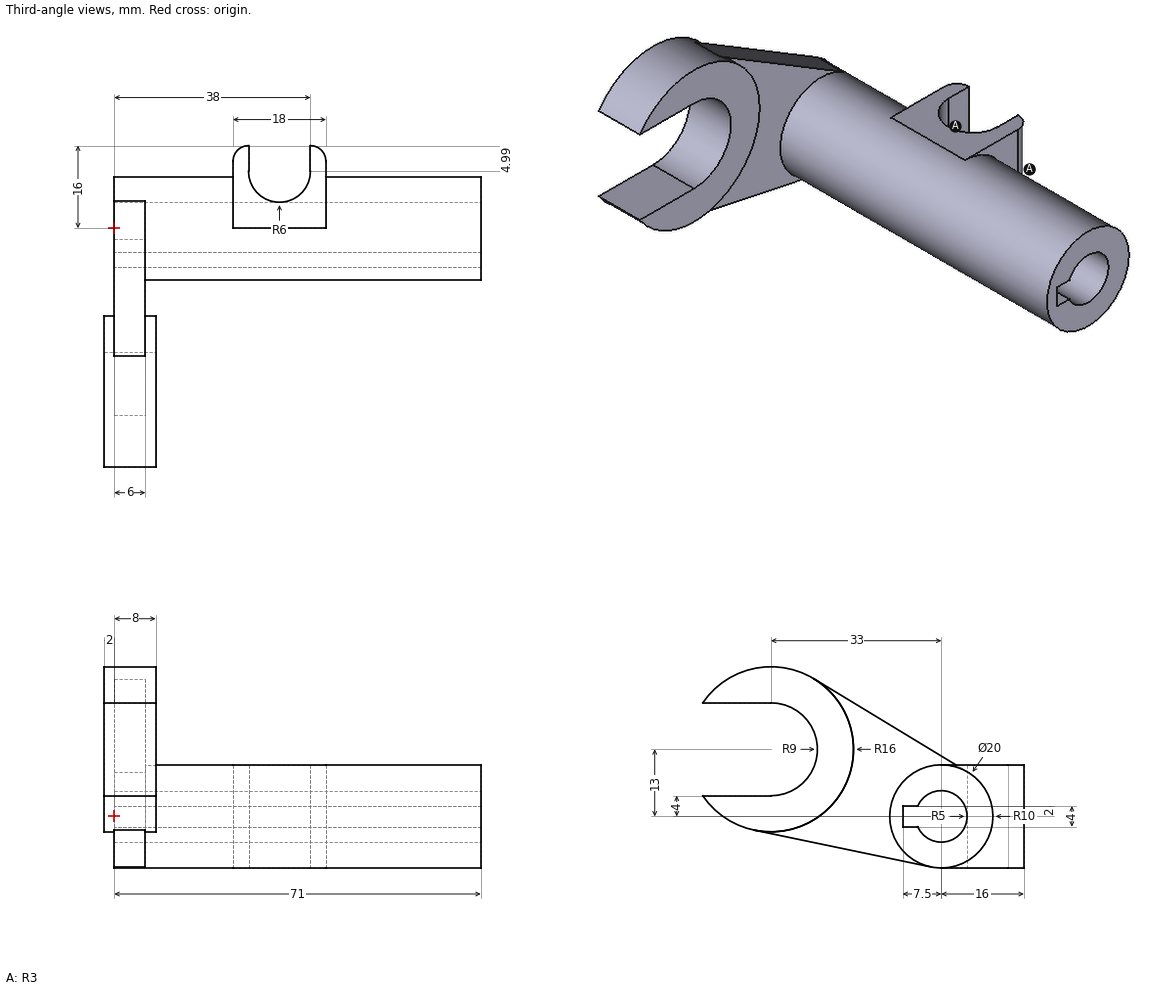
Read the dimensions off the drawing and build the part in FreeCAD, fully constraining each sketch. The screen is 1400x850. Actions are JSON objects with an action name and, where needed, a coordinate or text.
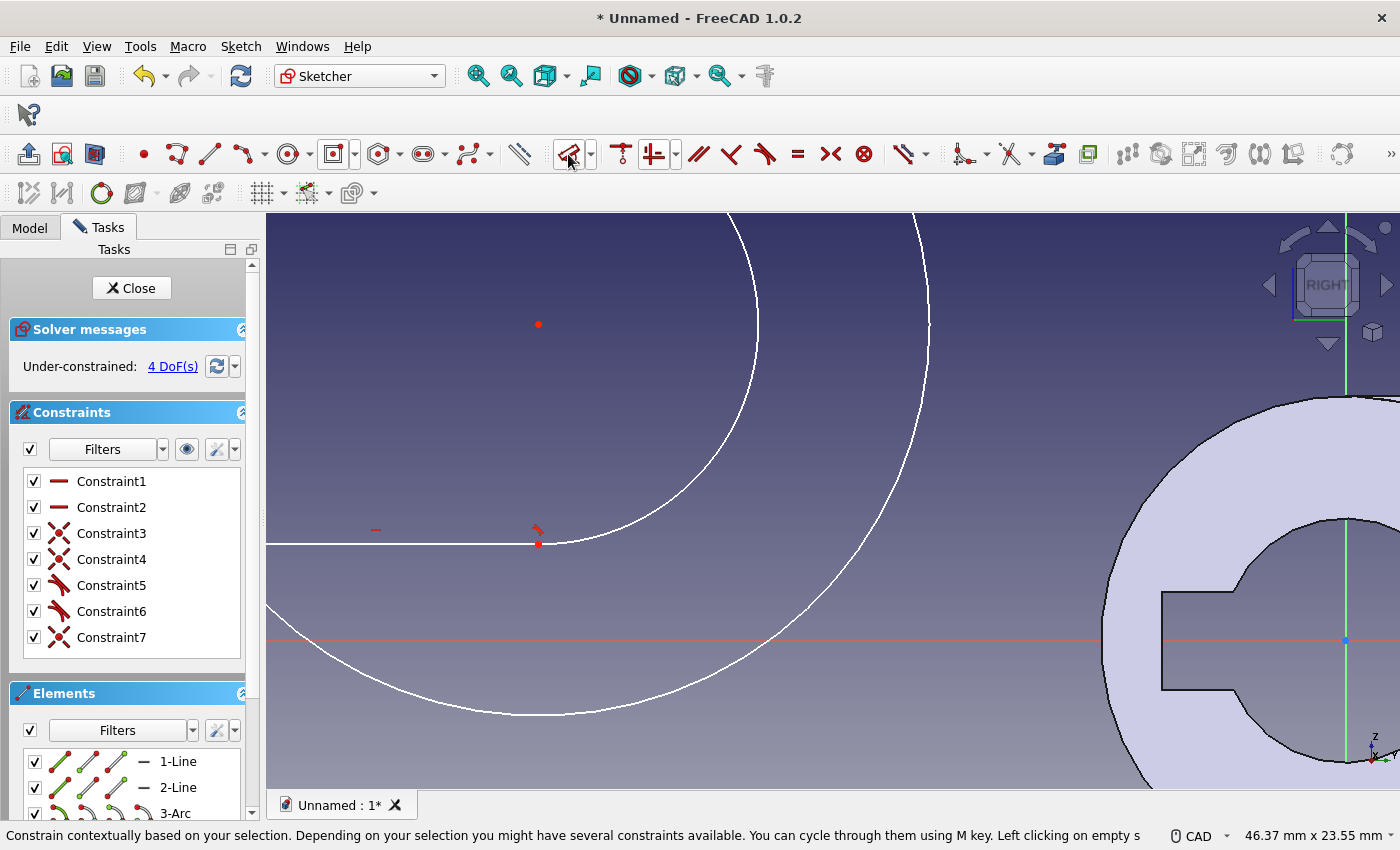
{"action": "left_click", "coordinate": [744, 658]}
{"action": "left_click", "coordinate": [761, 685]}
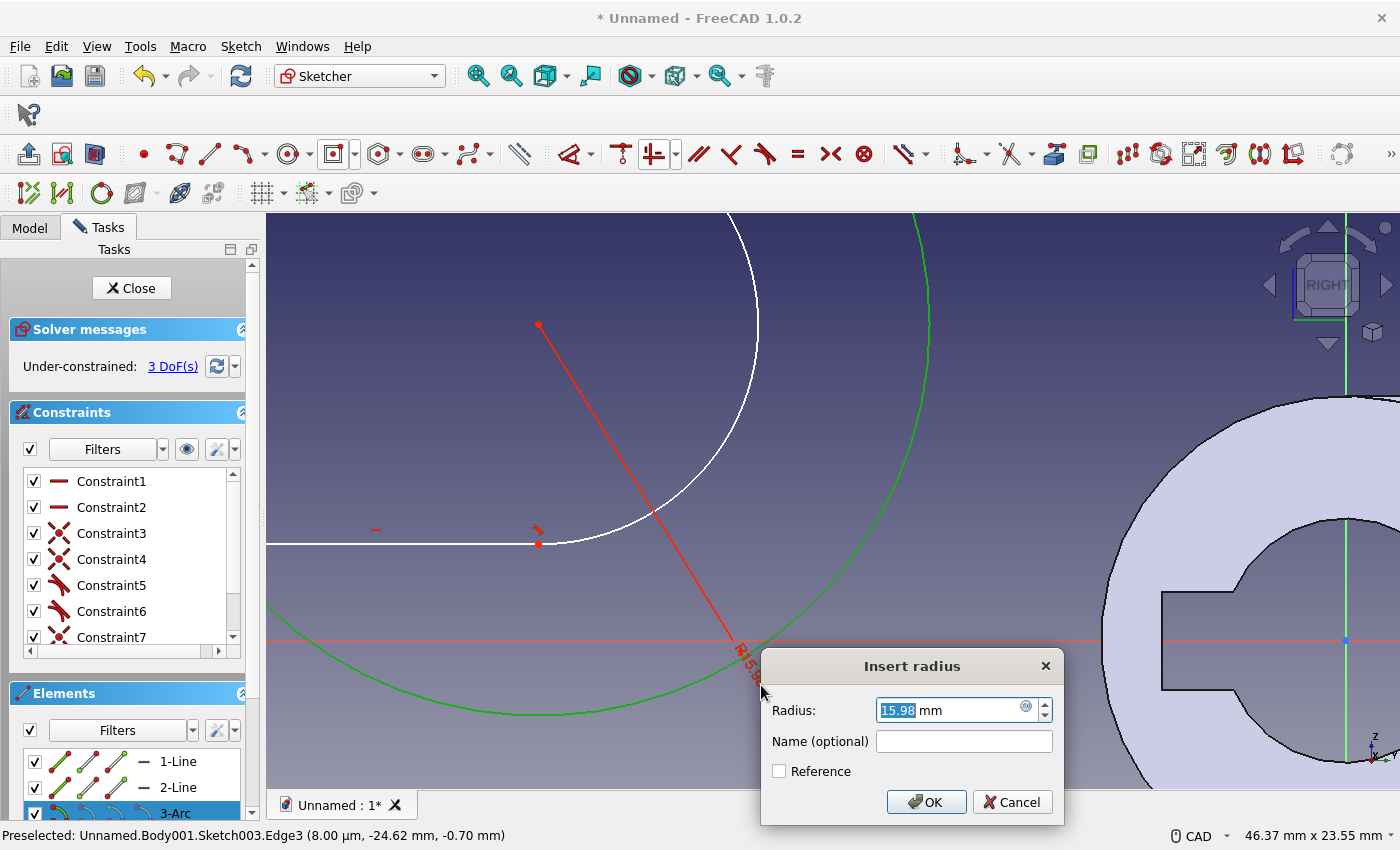
{"action": "type", "text": "16"}
{"action": "key", "text": "Return"}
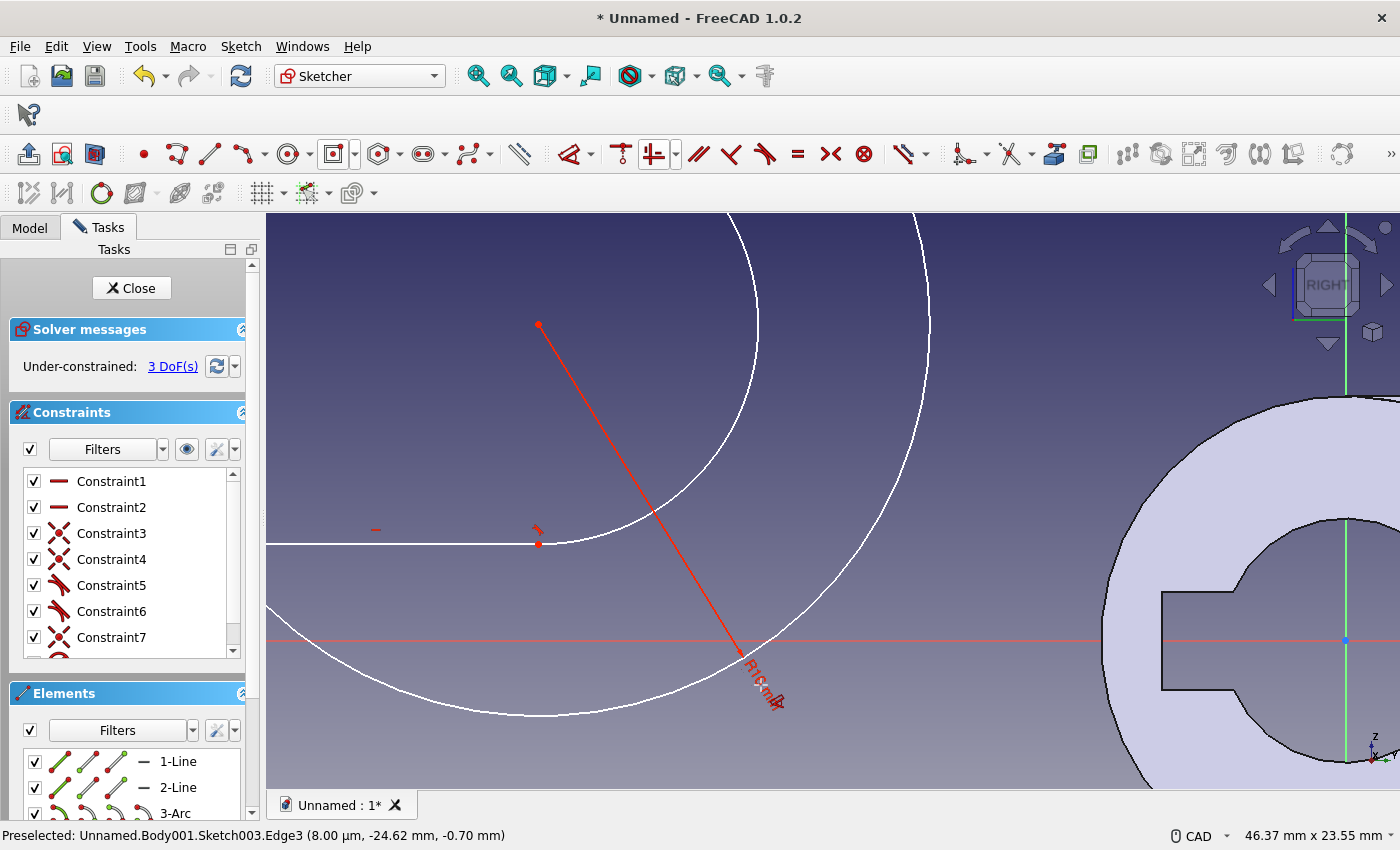
{"action": "left_click", "coordinate": [716, 454]}
{"action": "left_click", "coordinate": [742, 473]}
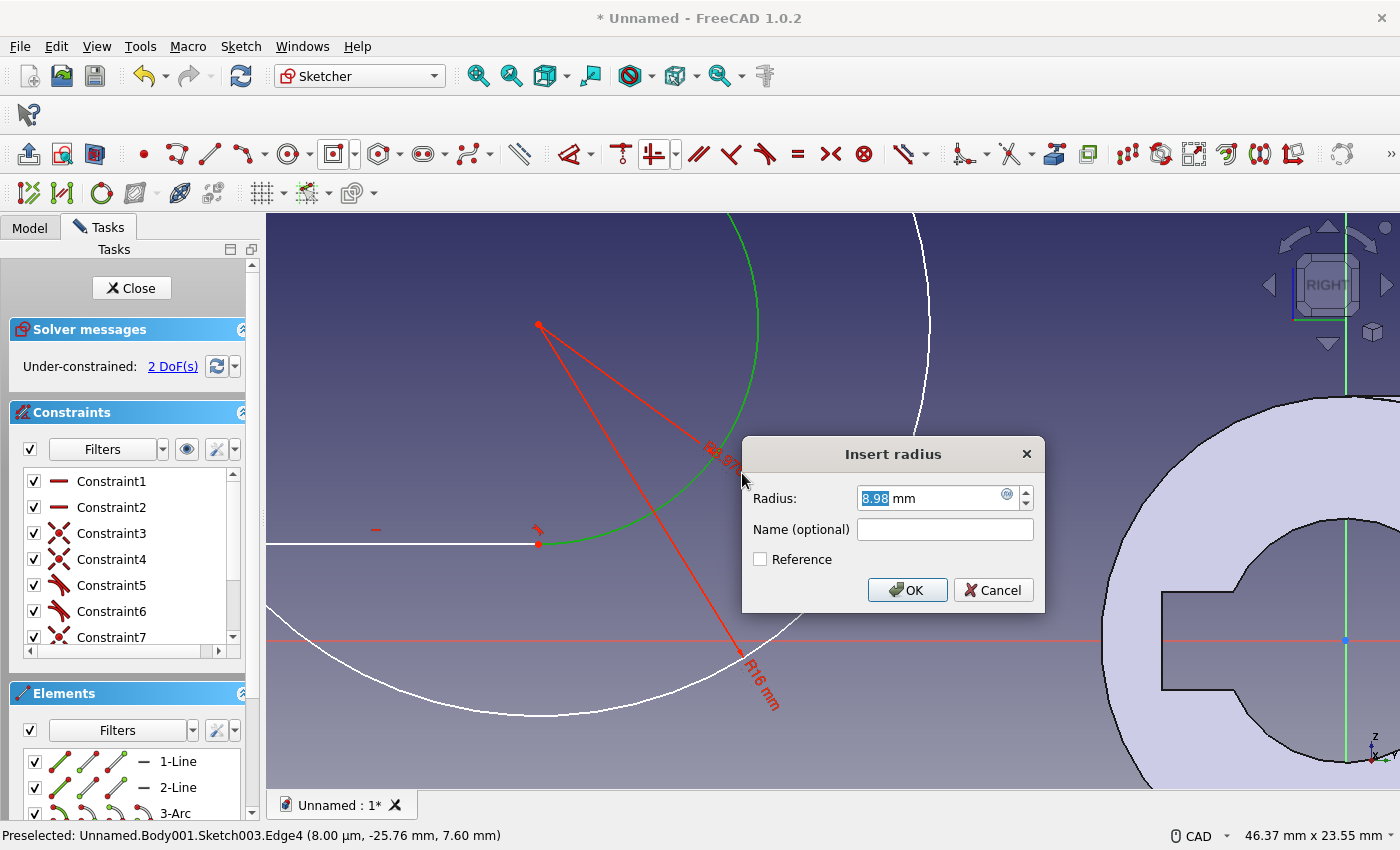
{"action": "type", "text": "9"}
{"action": "key", "text": "Return"}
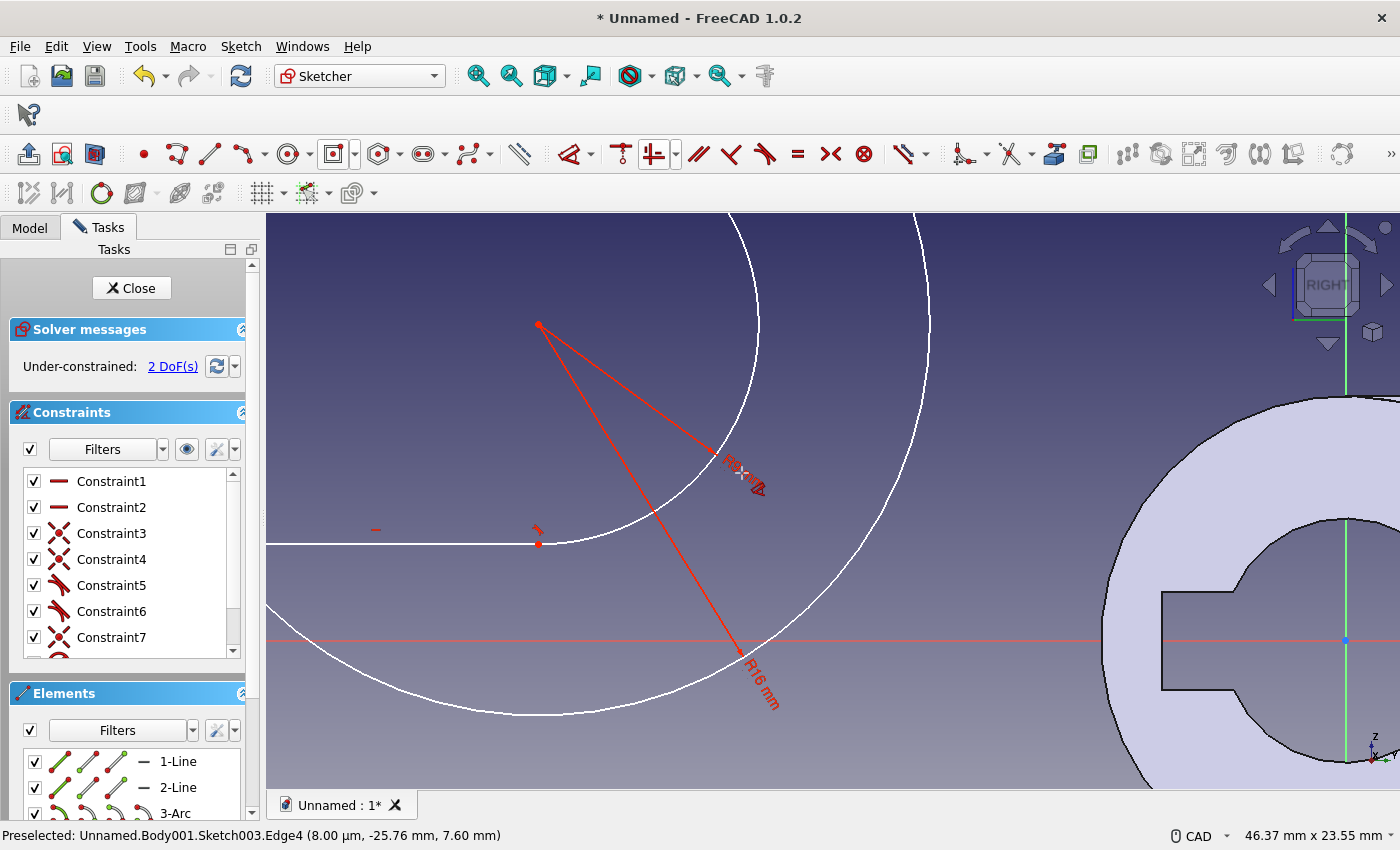
{"action": "scroll", "coordinate": [745, 658], "scroll_direction": "down", "scroll_amount": 3}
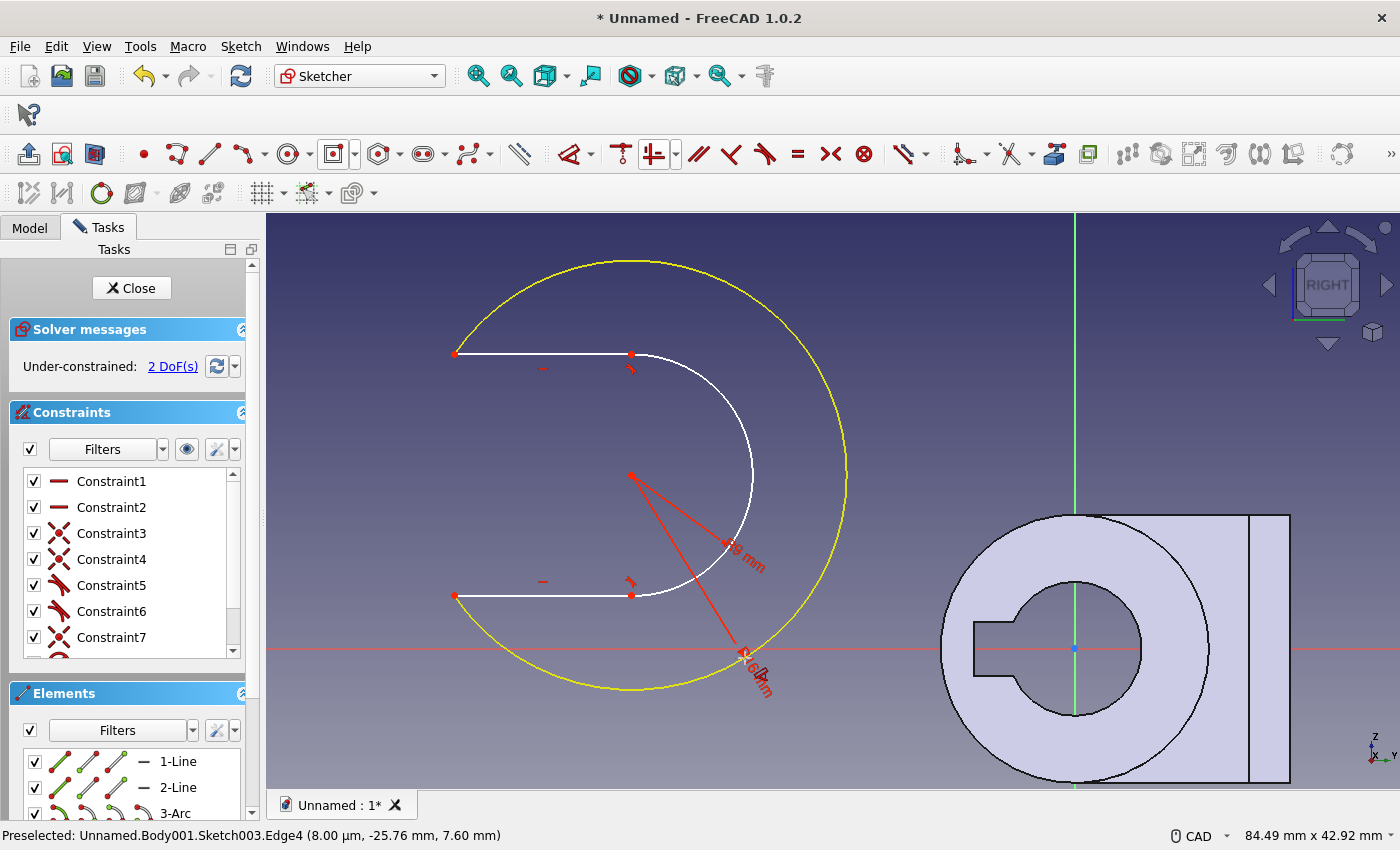
{"action": "left_click", "coordinate": [454, 596]}
{"action": "left_click", "coordinate": [1109, 622]}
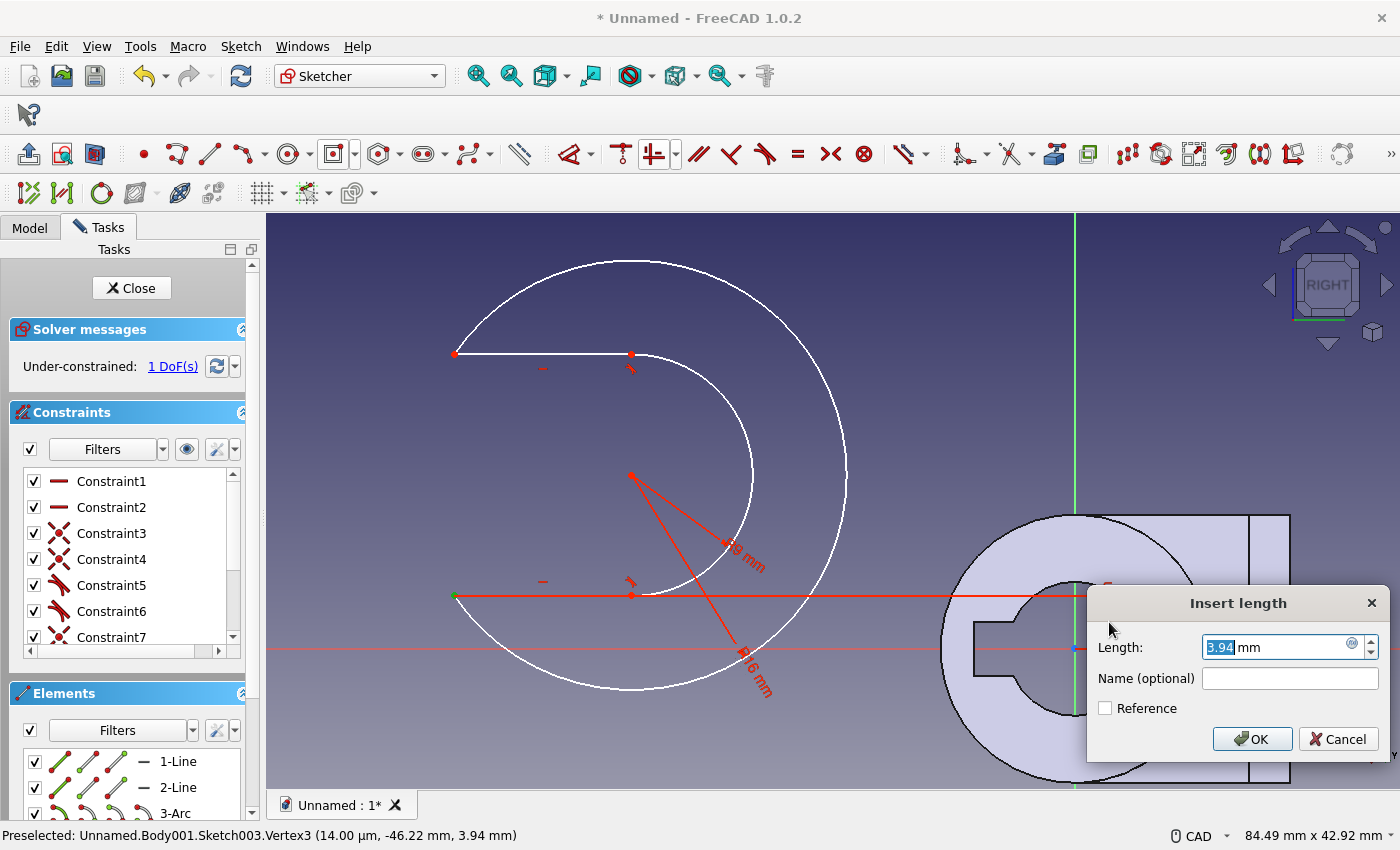
{"action": "type", "text": "4"}
{"action": "key", "text": "Return"}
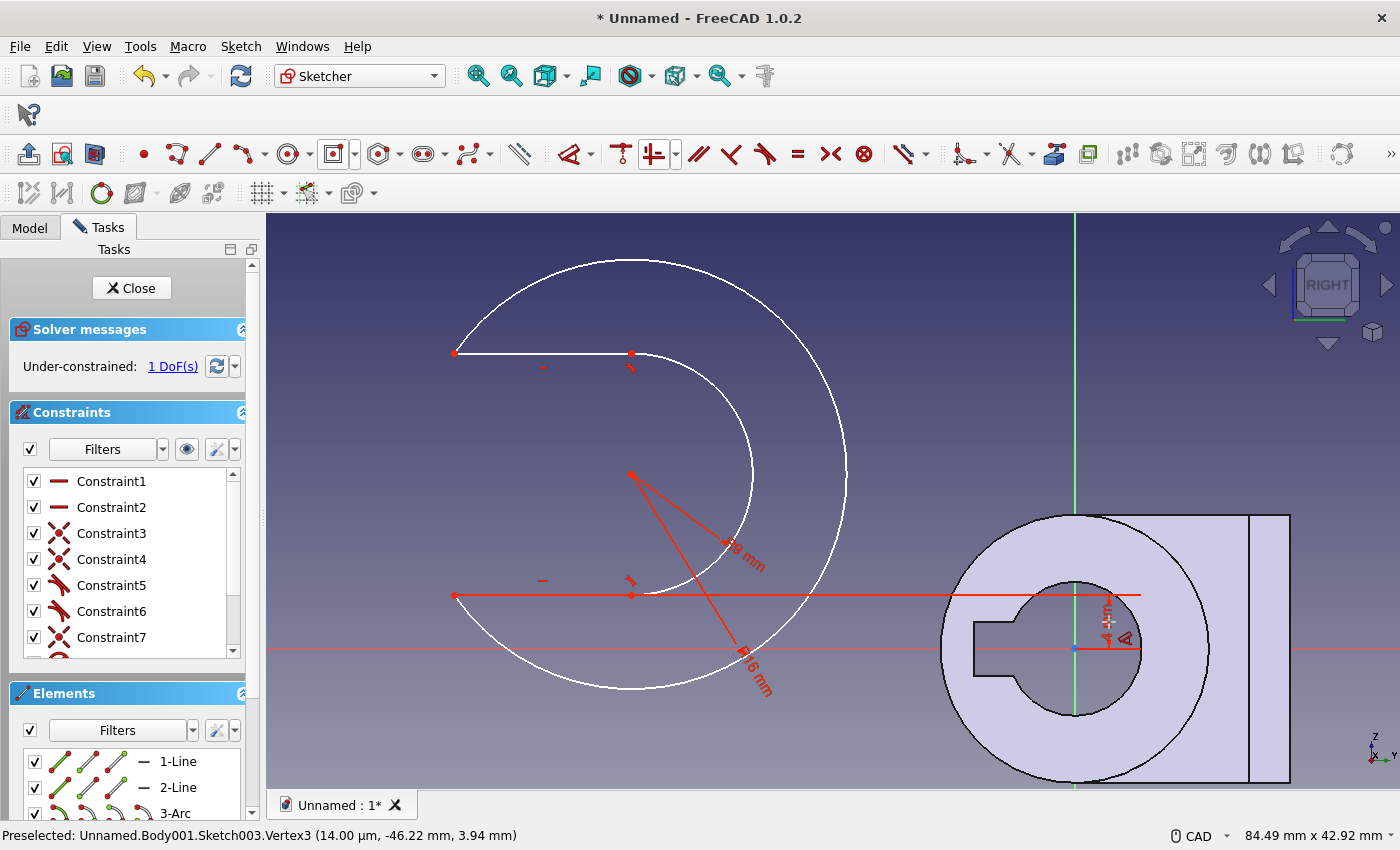
{"action": "left_click", "coordinate": [632, 354]}
{"action": "left_click", "coordinate": [853, 683]}